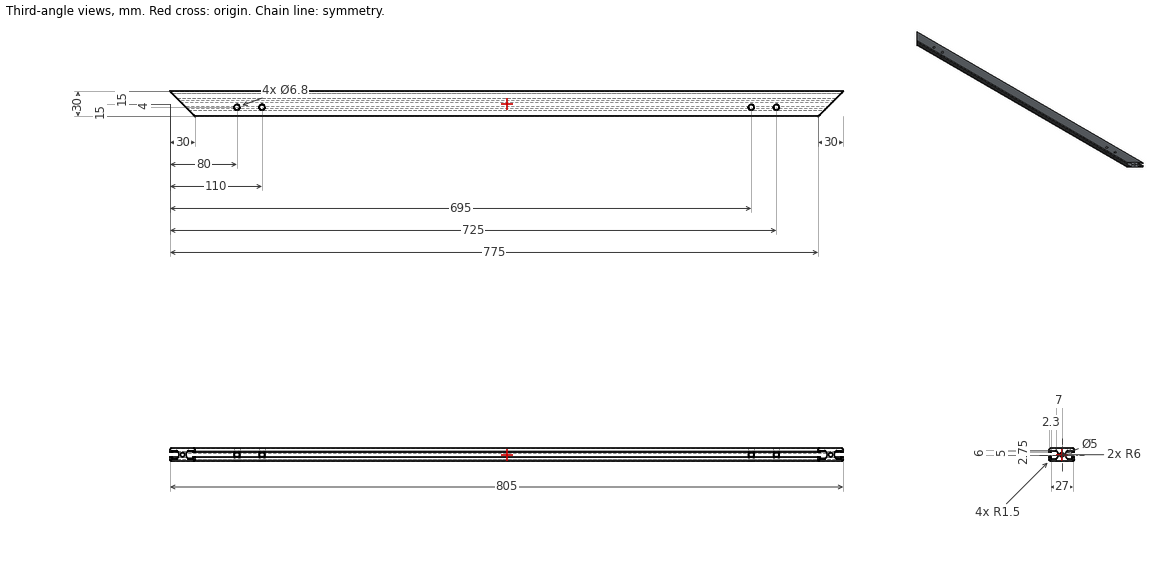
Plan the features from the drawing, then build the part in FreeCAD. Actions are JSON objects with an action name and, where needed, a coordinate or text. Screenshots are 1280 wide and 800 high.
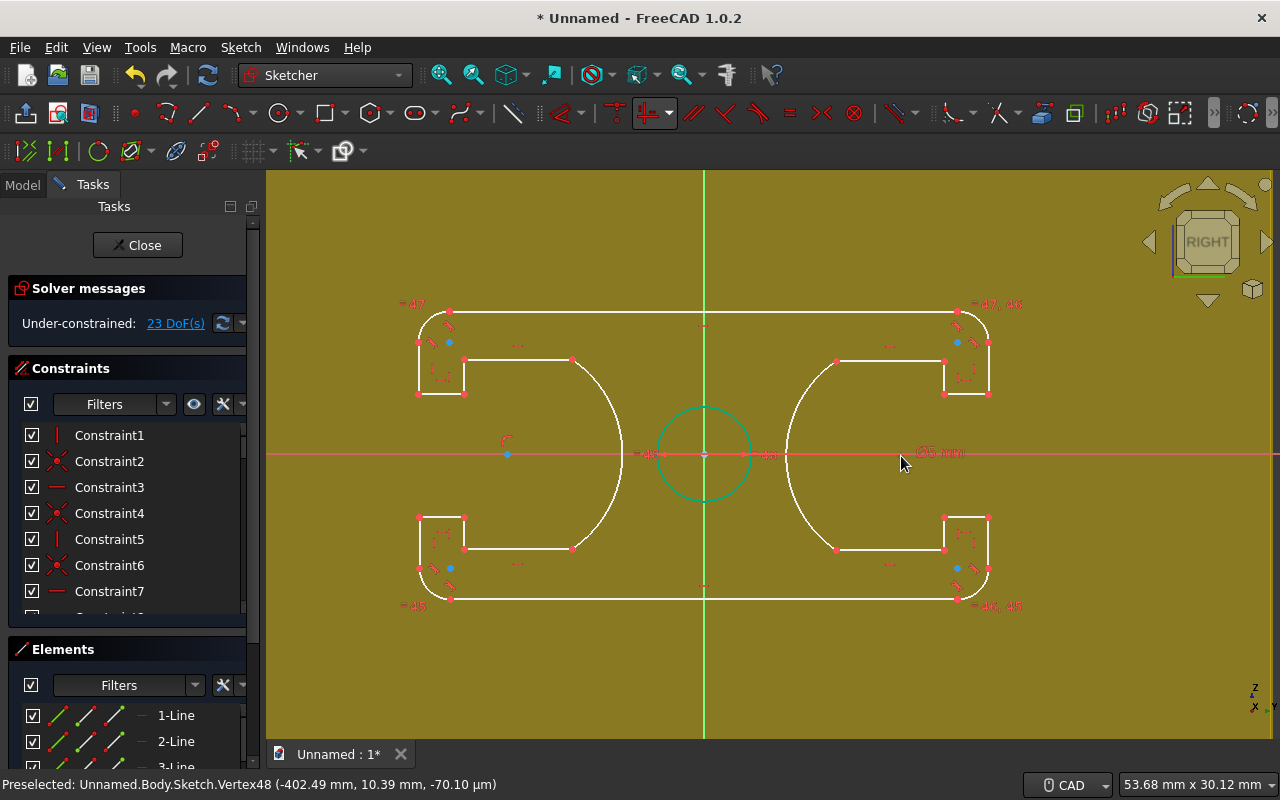
{"action": "left_click", "coordinate": [353, 454]}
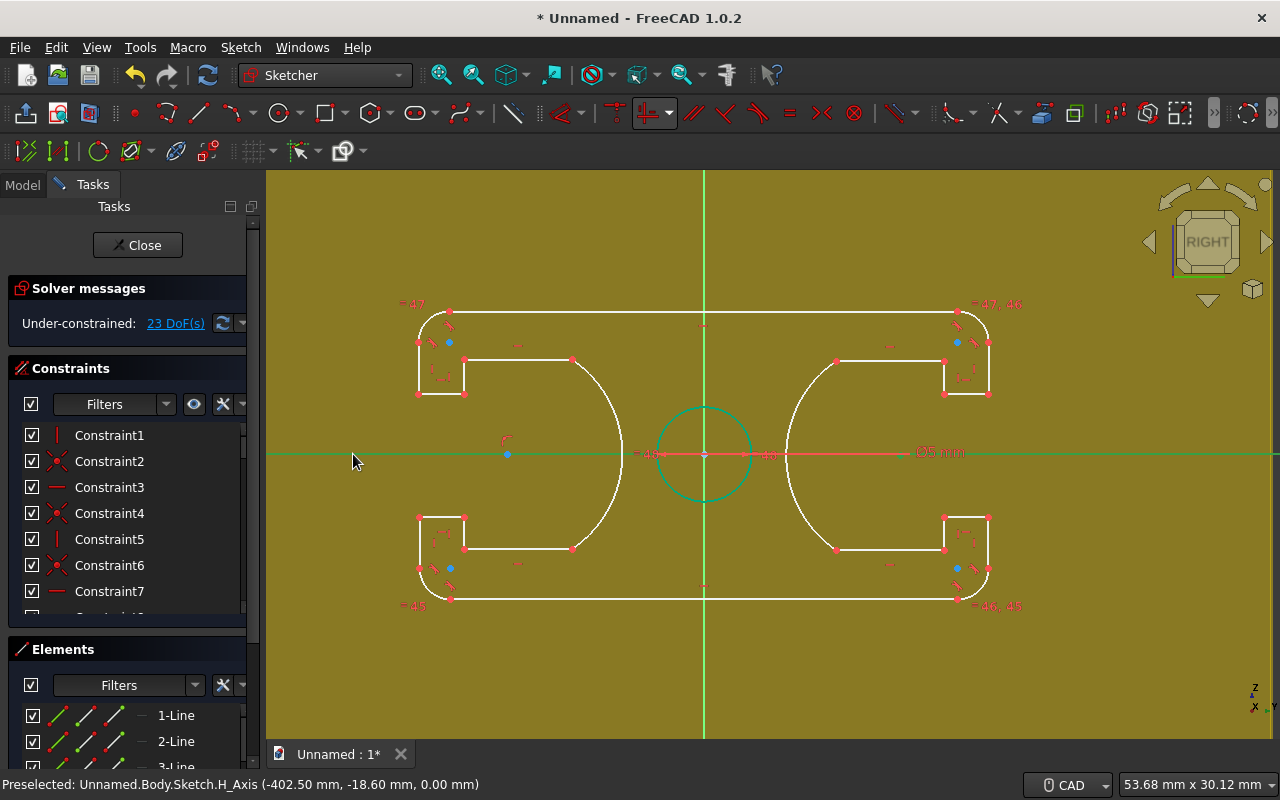
{"action": "left_click", "coordinate": [616, 114]}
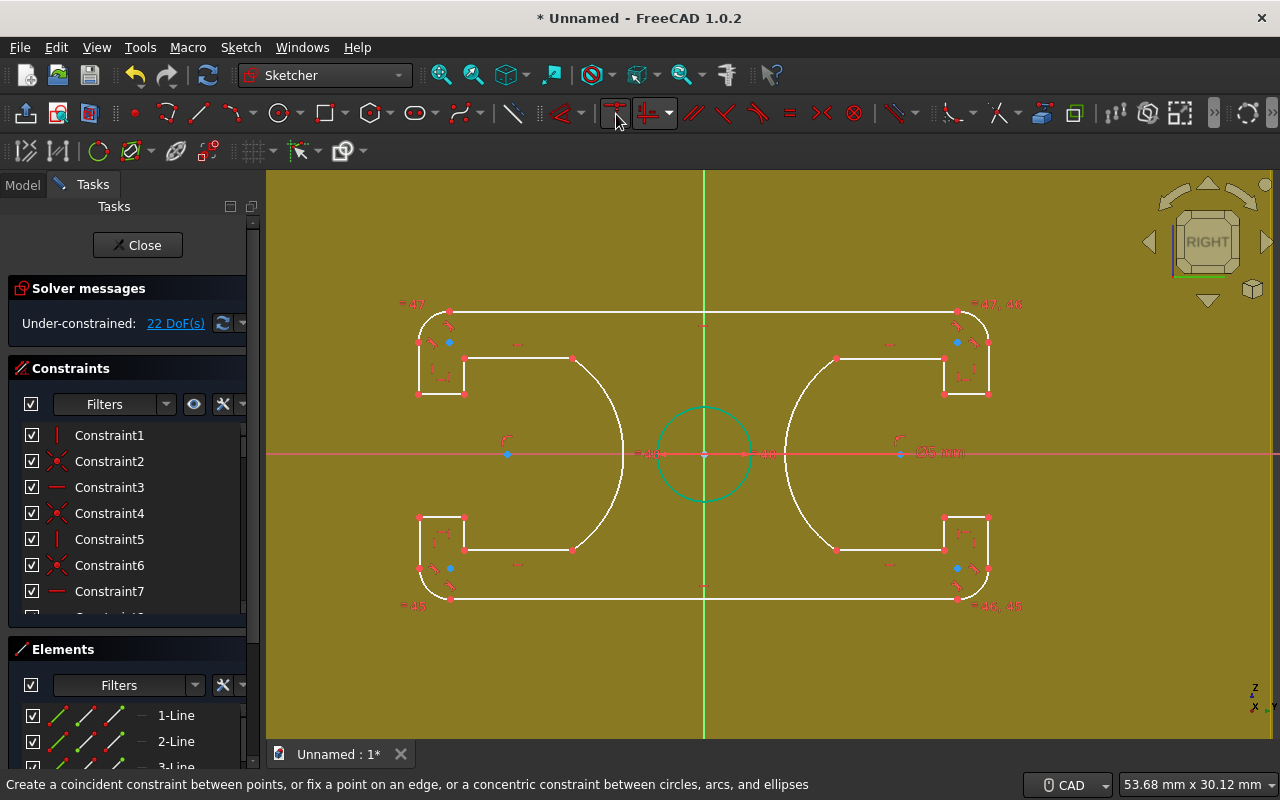
{"action": "left_click", "coordinate": [958, 569]}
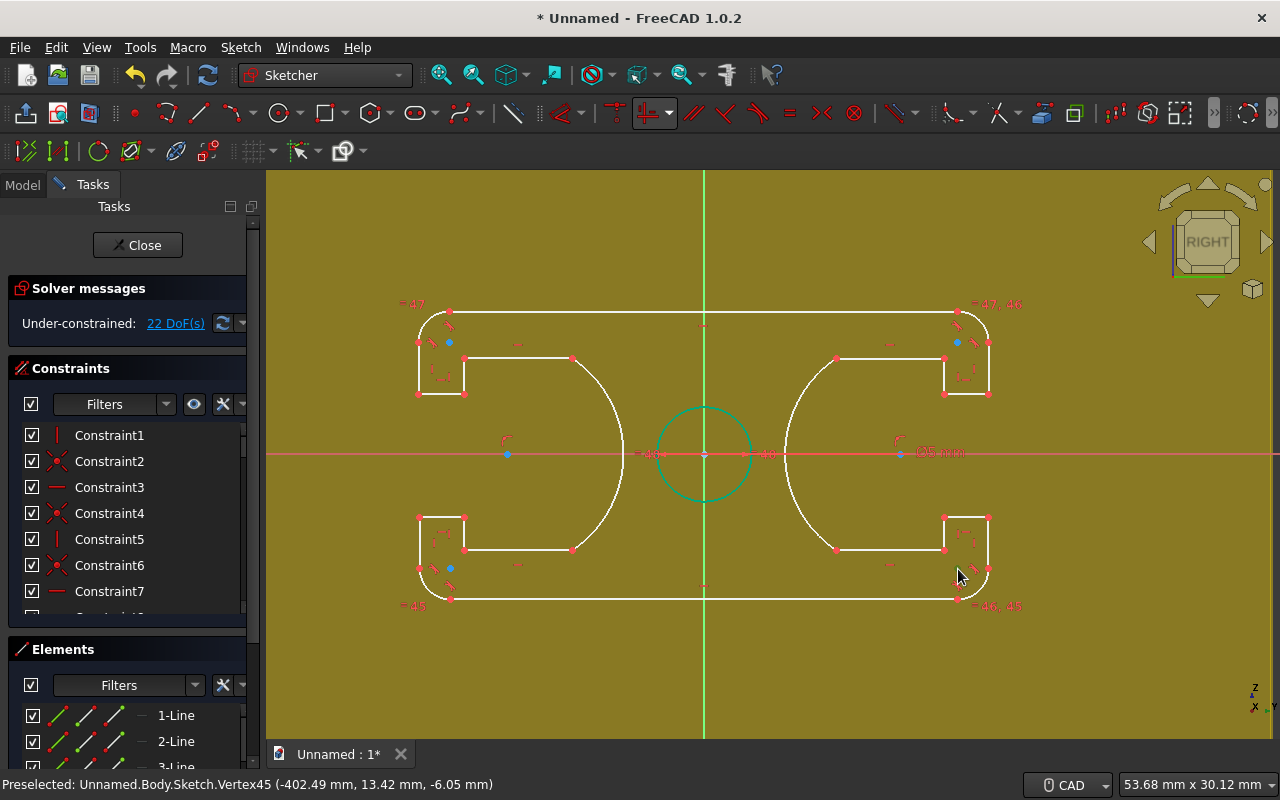
{"action": "left_click", "coordinate": [958, 342]}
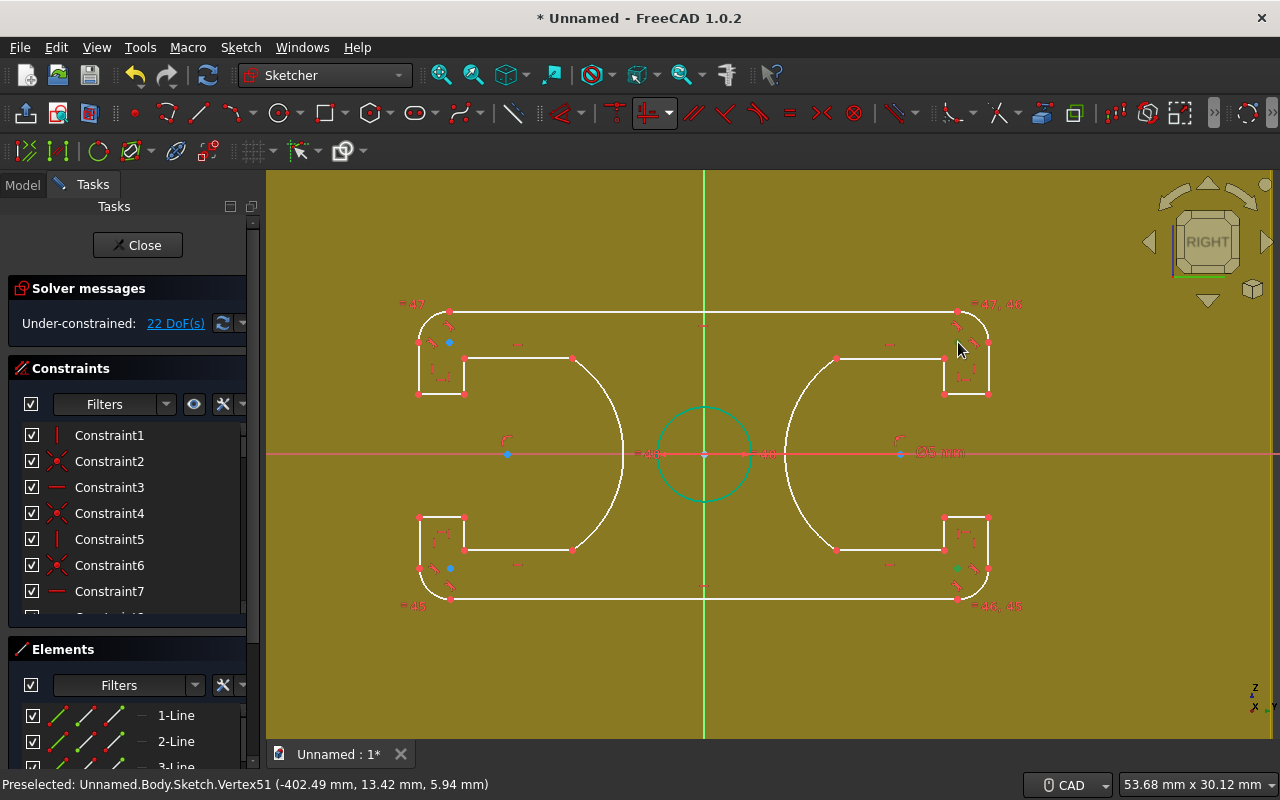
{"action": "left_click", "coordinate": [353, 454]}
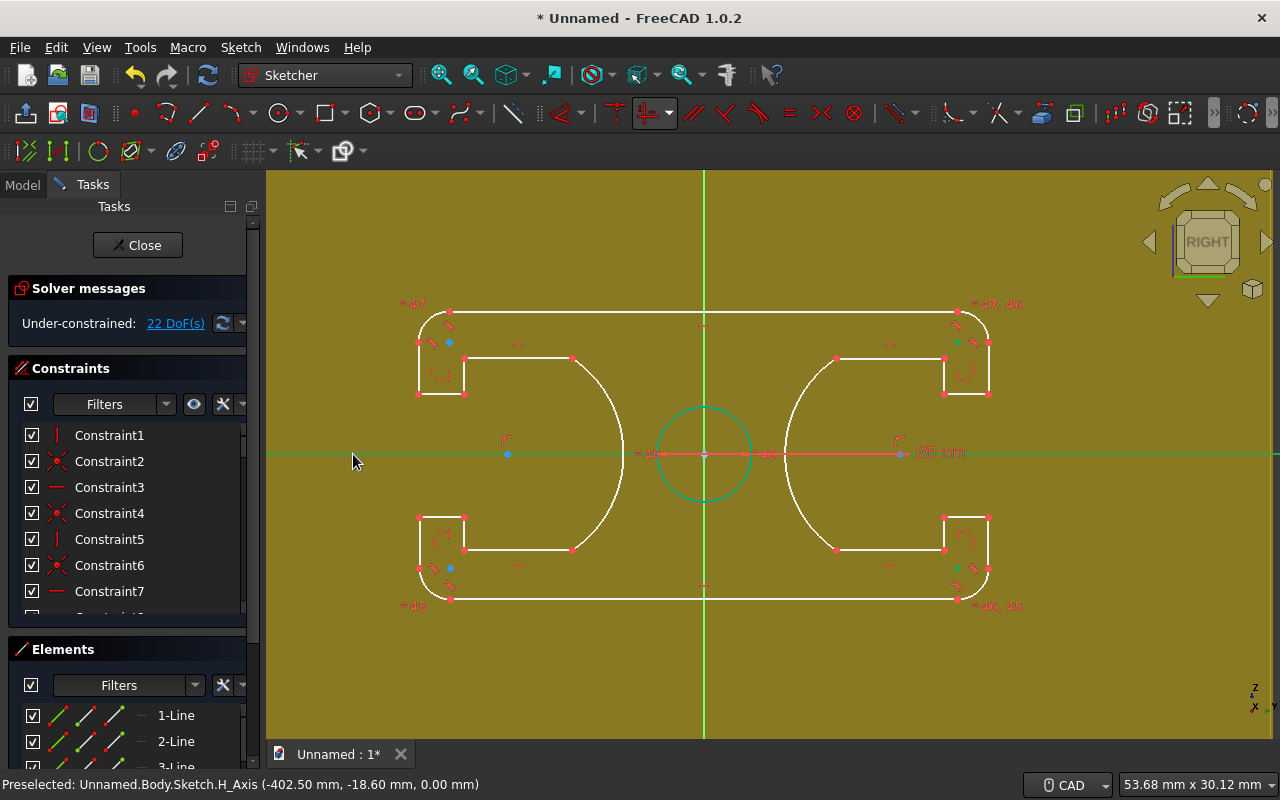
{"action": "left_click", "coordinate": [822, 114]}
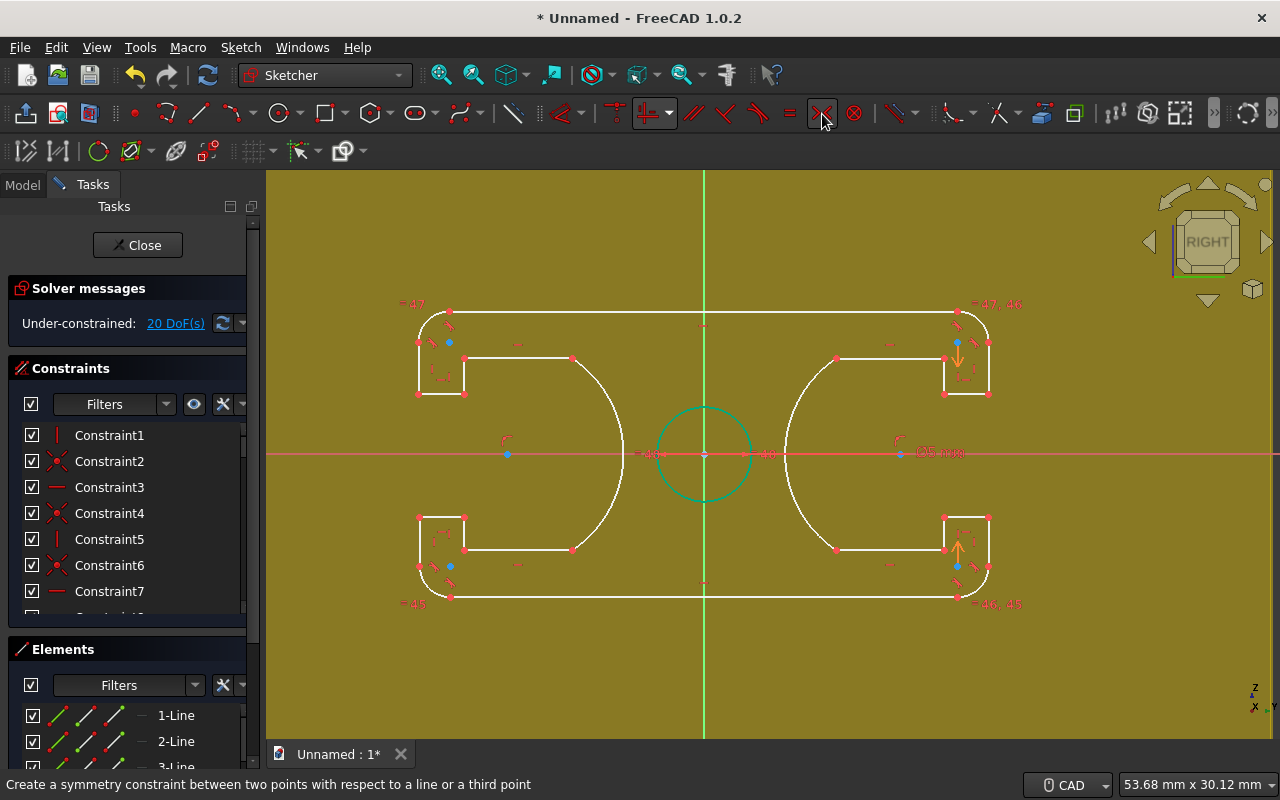
{"action": "left_click", "coordinate": [464, 358]}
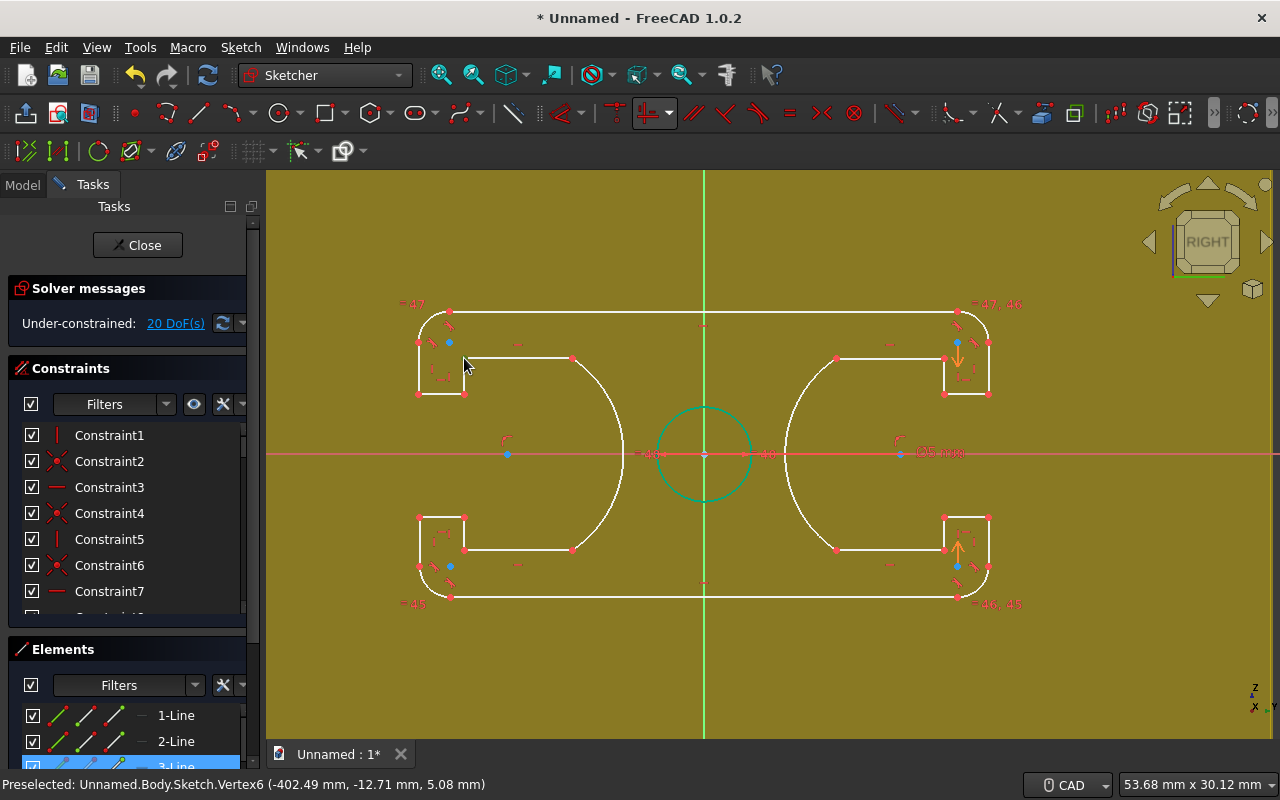
{"action": "left_click", "coordinate": [464, 550]}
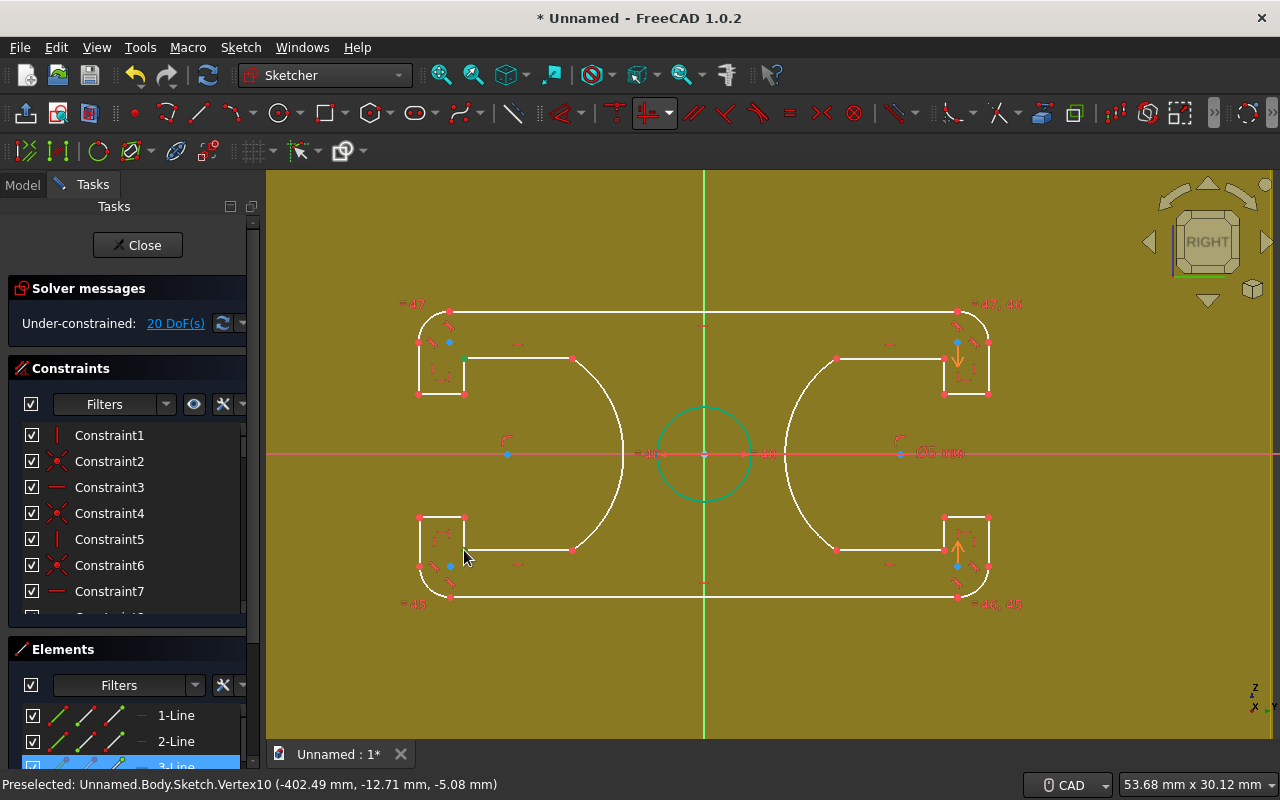
{"action": "left_click", "coordinate": [353, 454]}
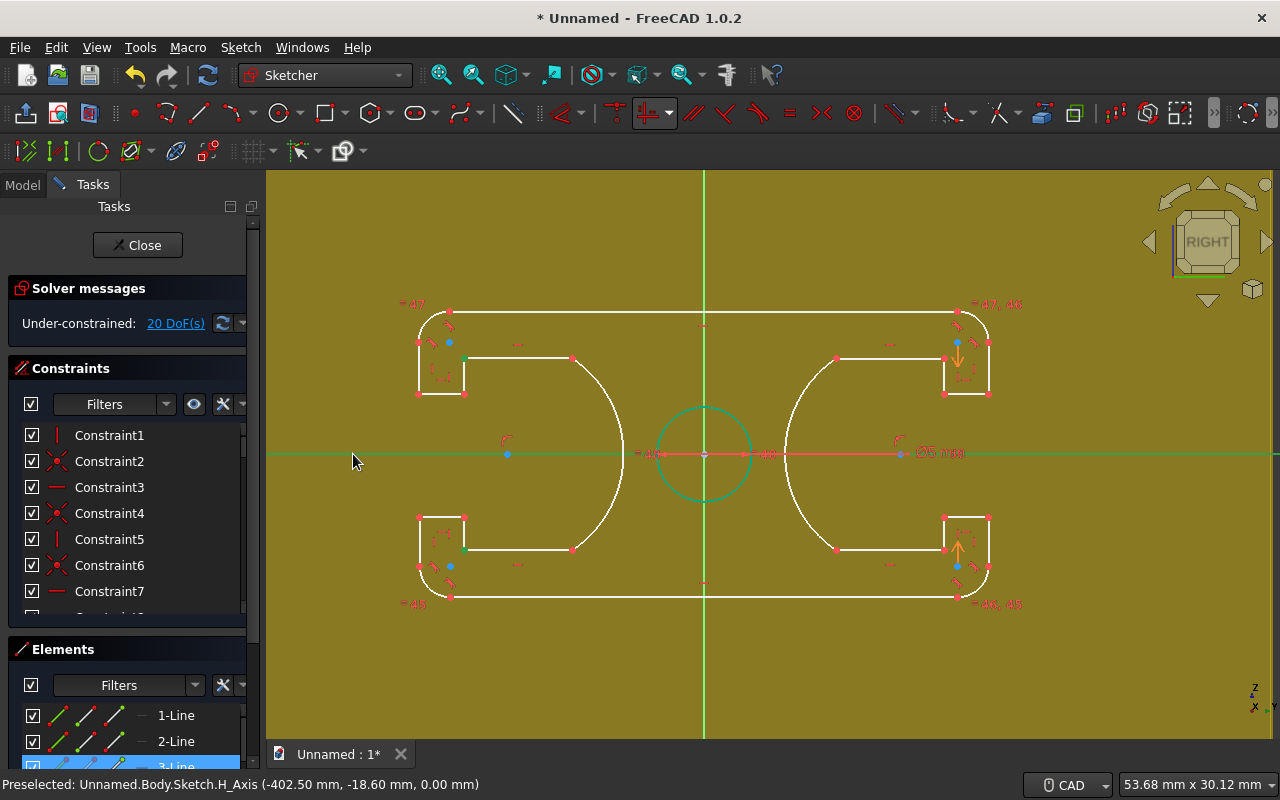
{"action": "left_click", "coordinate": [822, 114]}